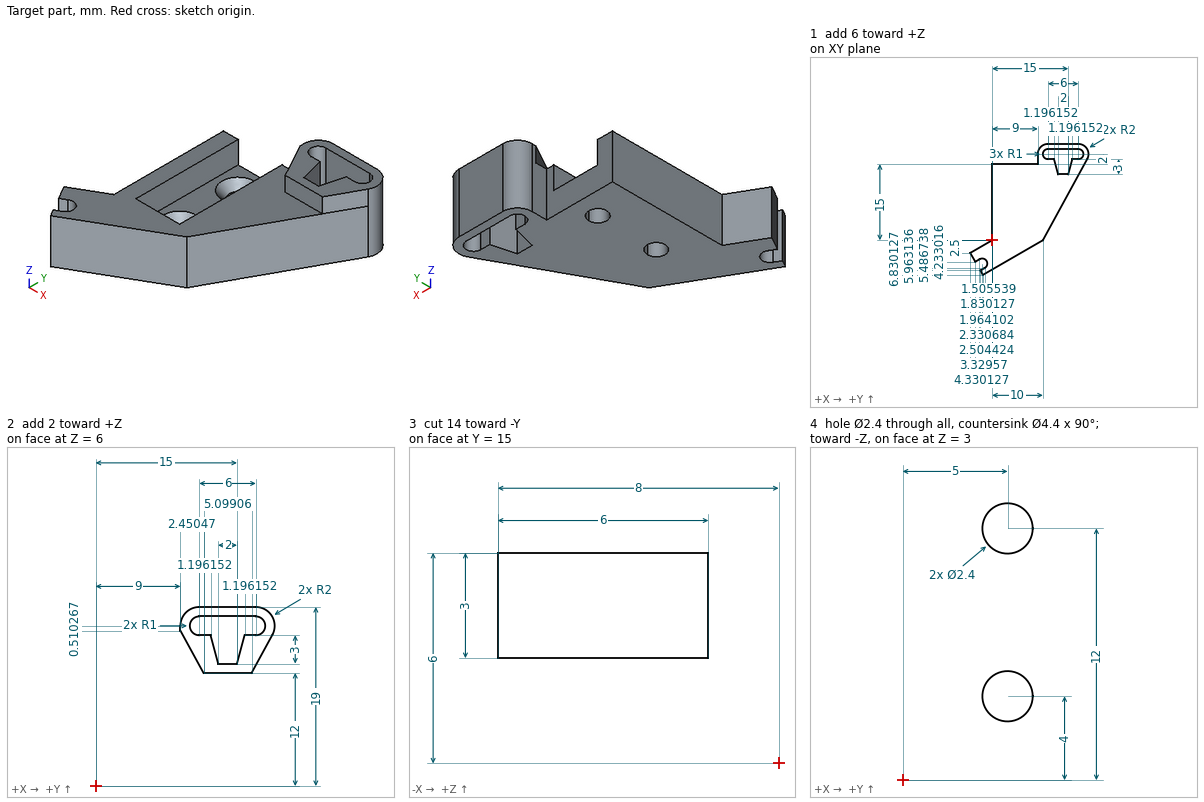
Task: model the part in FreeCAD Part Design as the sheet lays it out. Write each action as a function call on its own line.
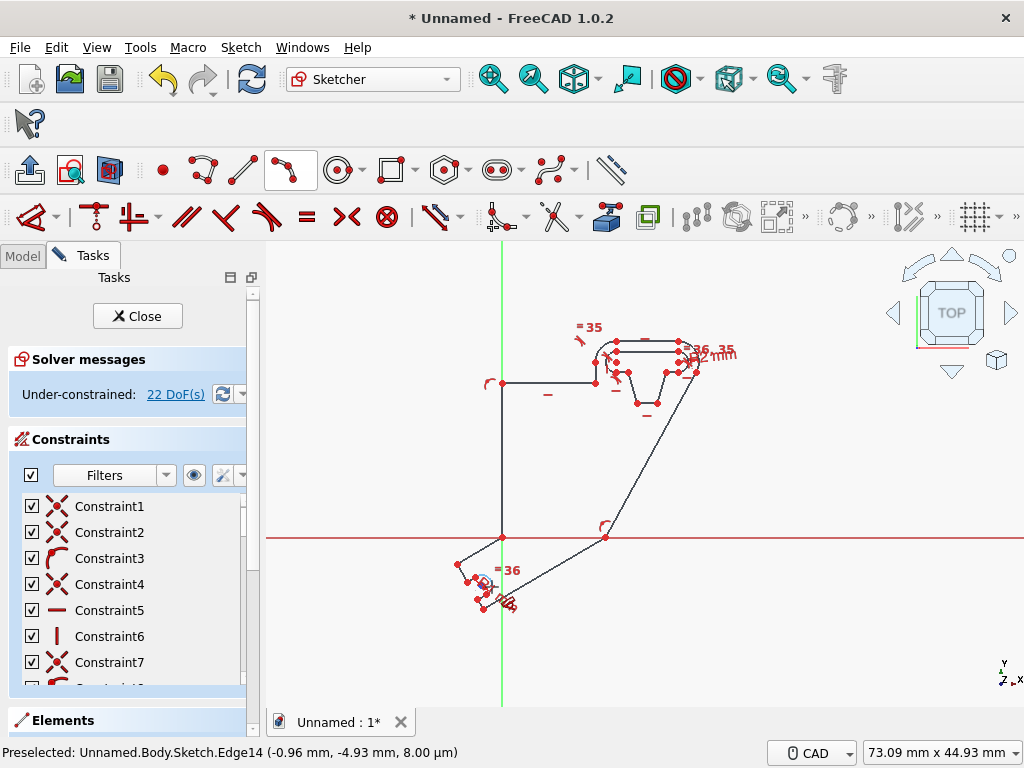
scroll(660, 341, up, 2)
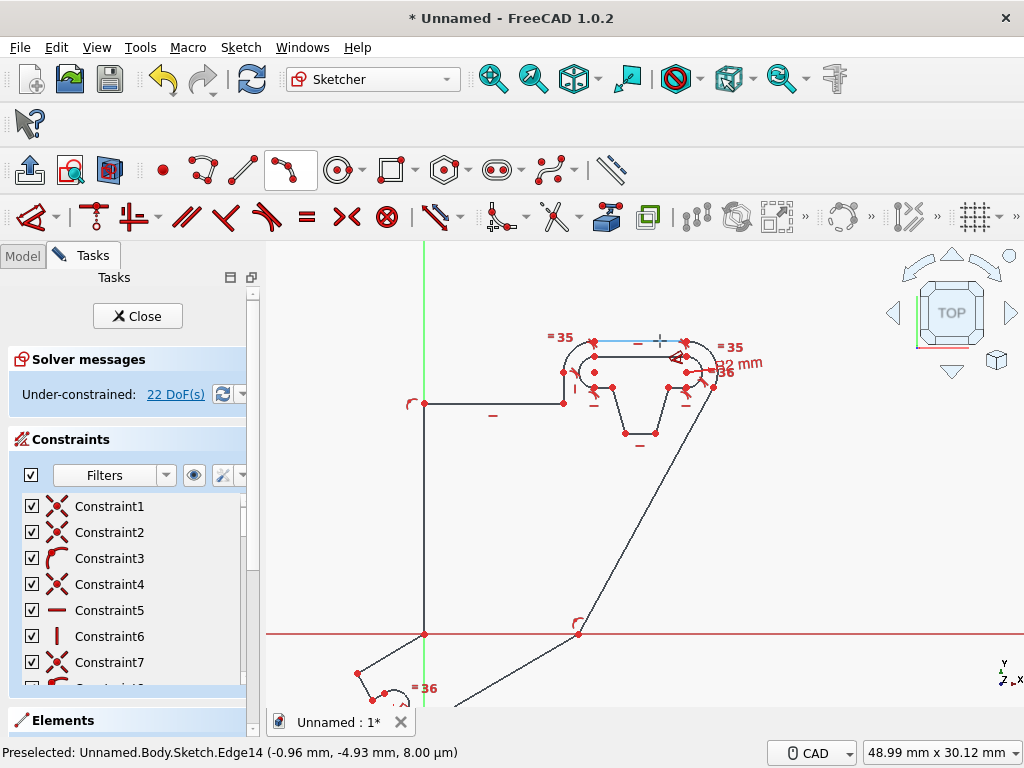
click(659, 341)
click(641, 307)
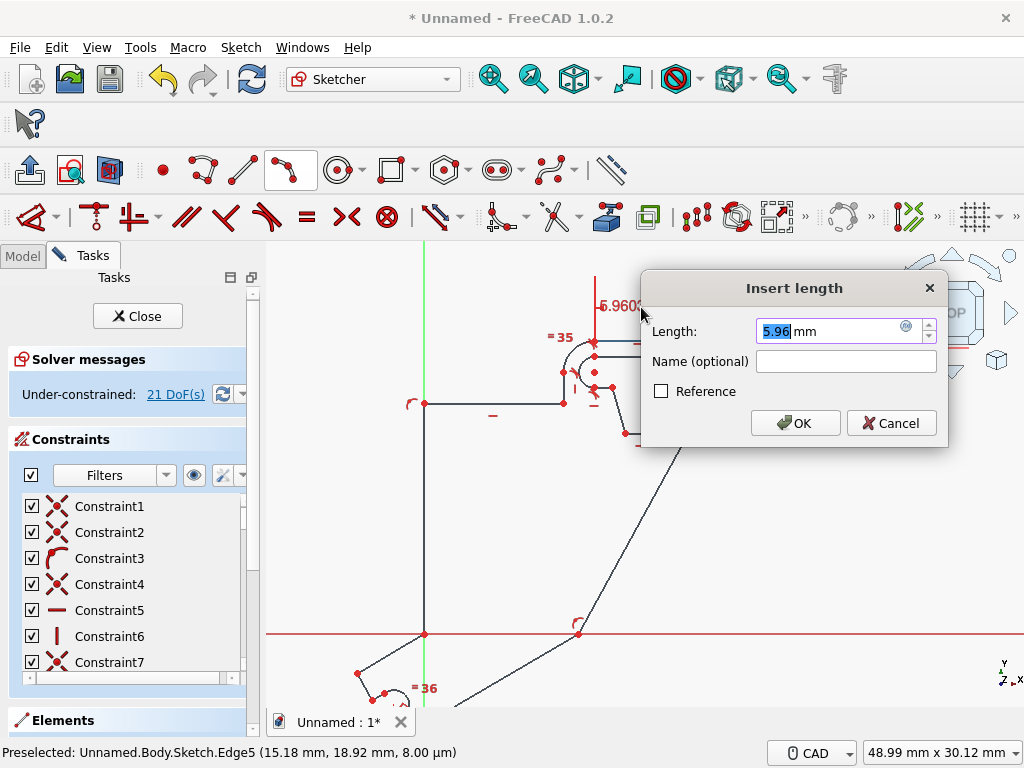
text(6)
key(Return)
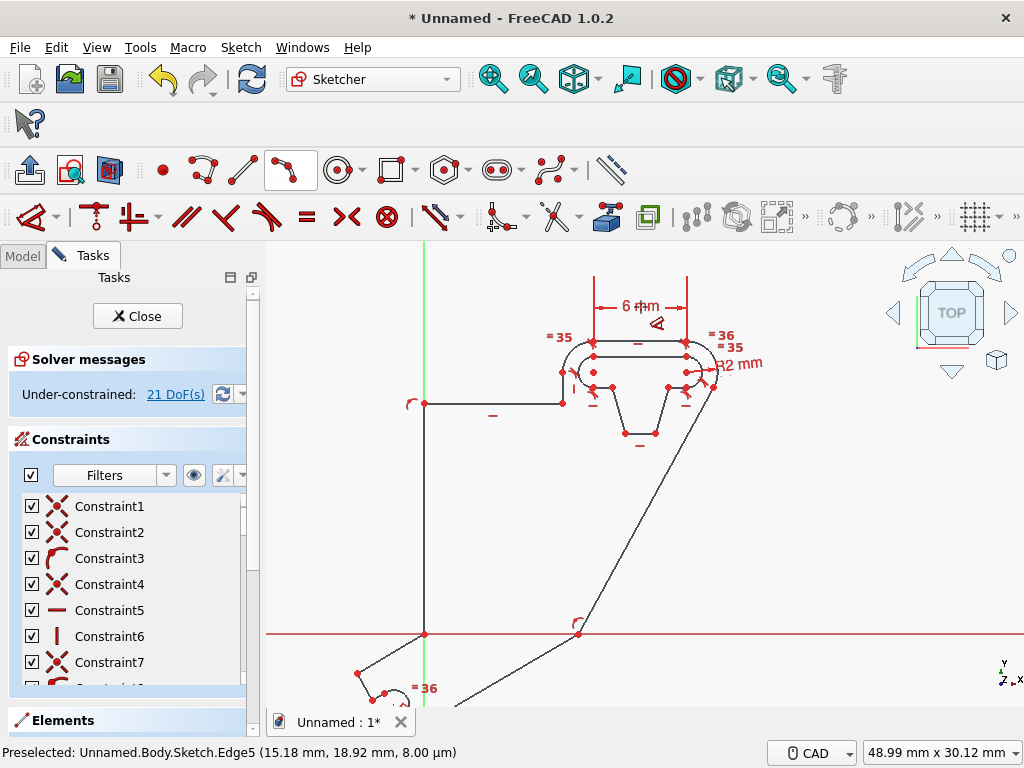
scroll(563, 382, up, 2)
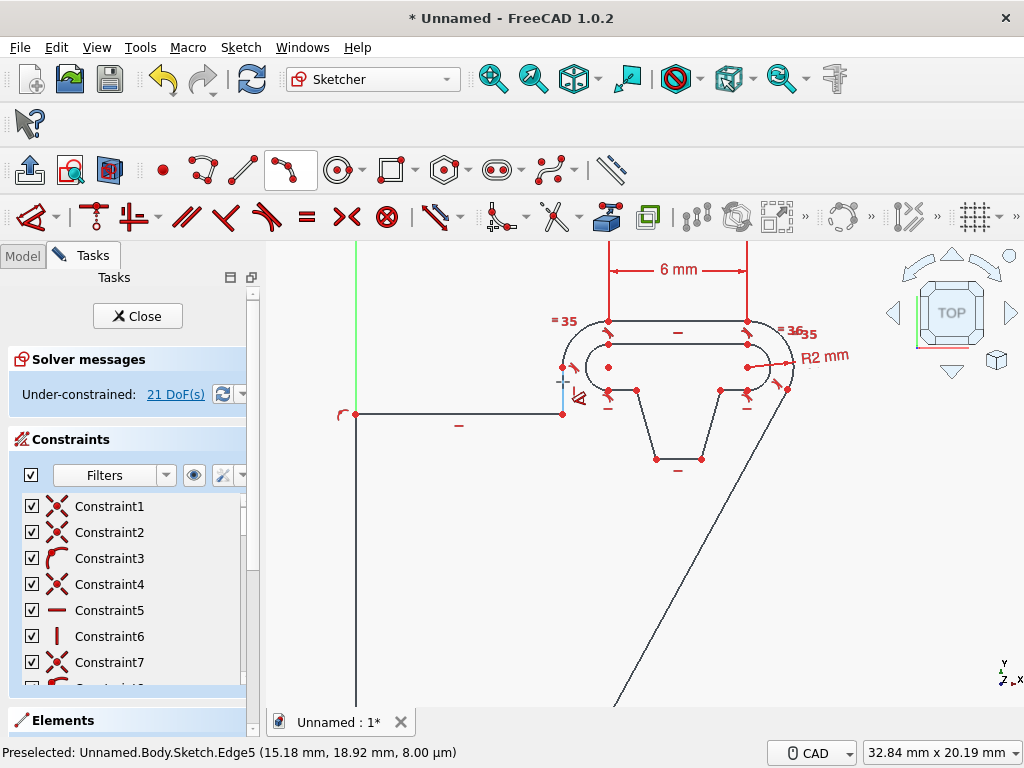
click(563, 381)
click(597, 402)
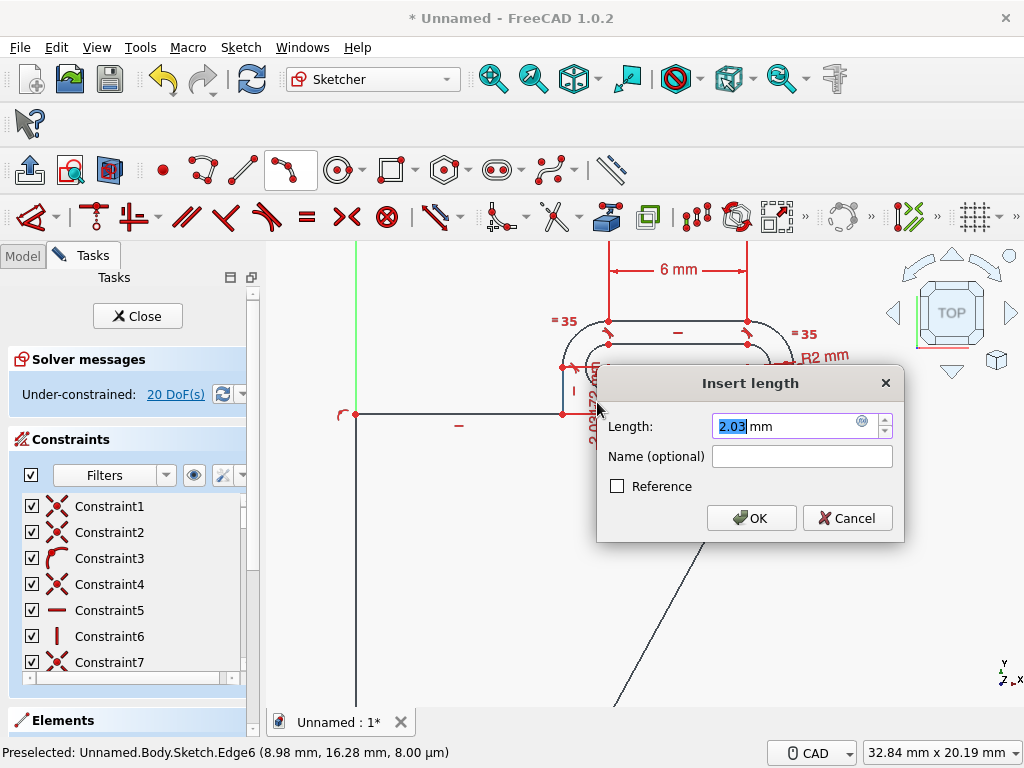
text(2)
key(Return)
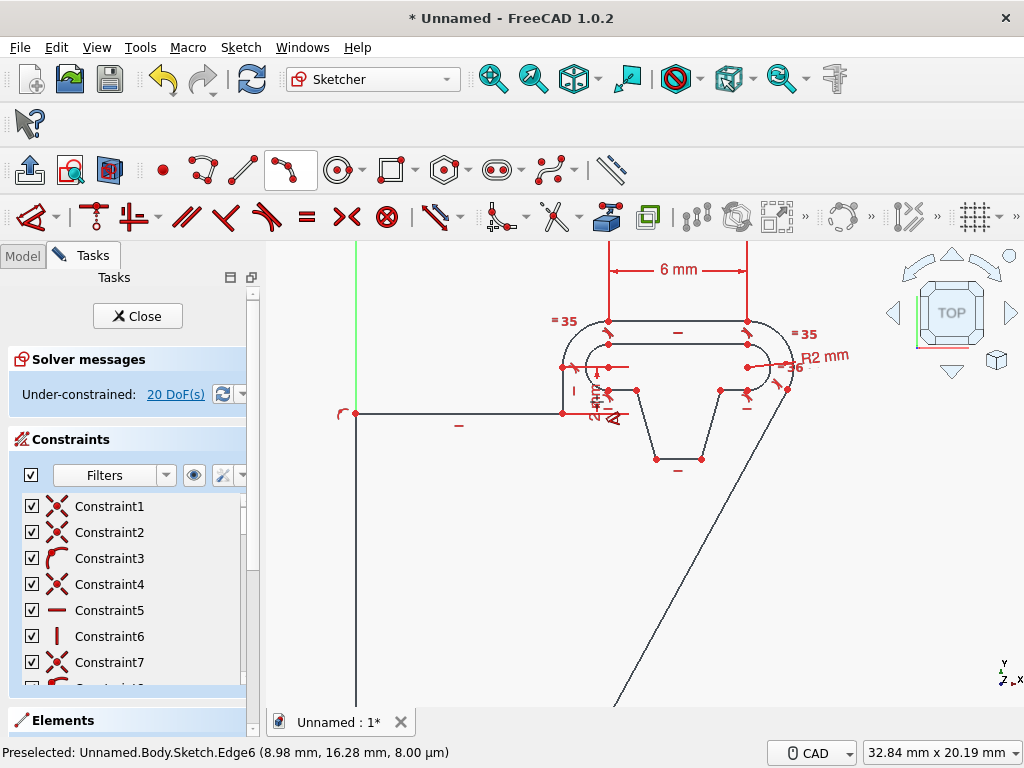
click(501, 414)
click(459, 380)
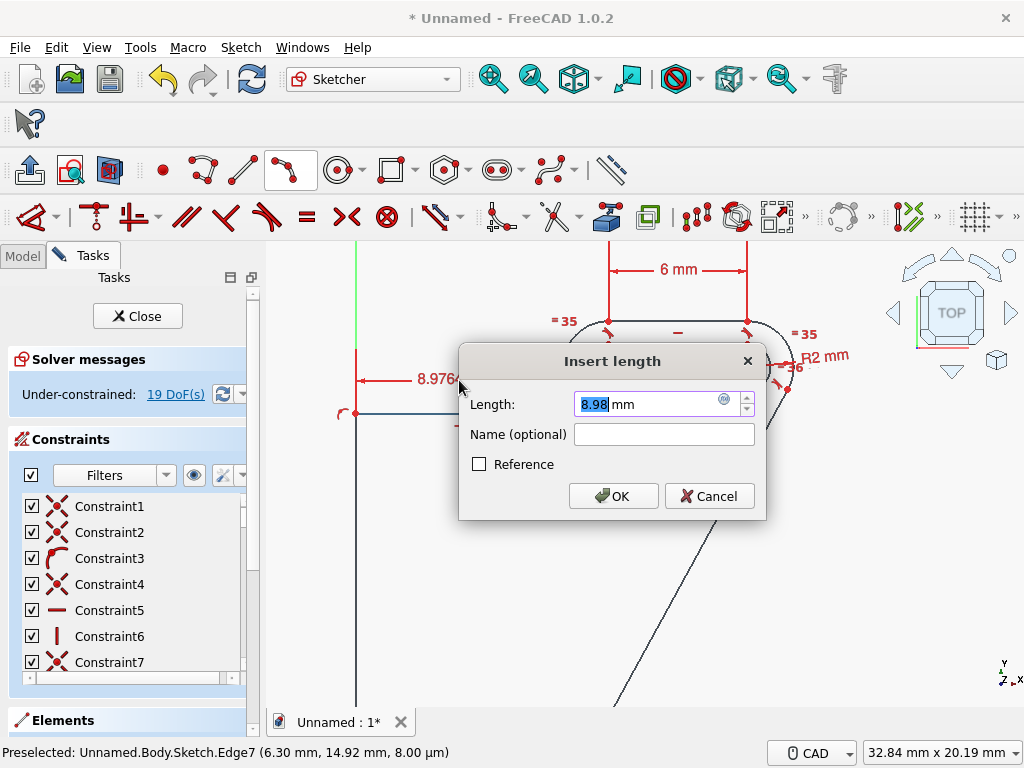
text(9)
key(Return)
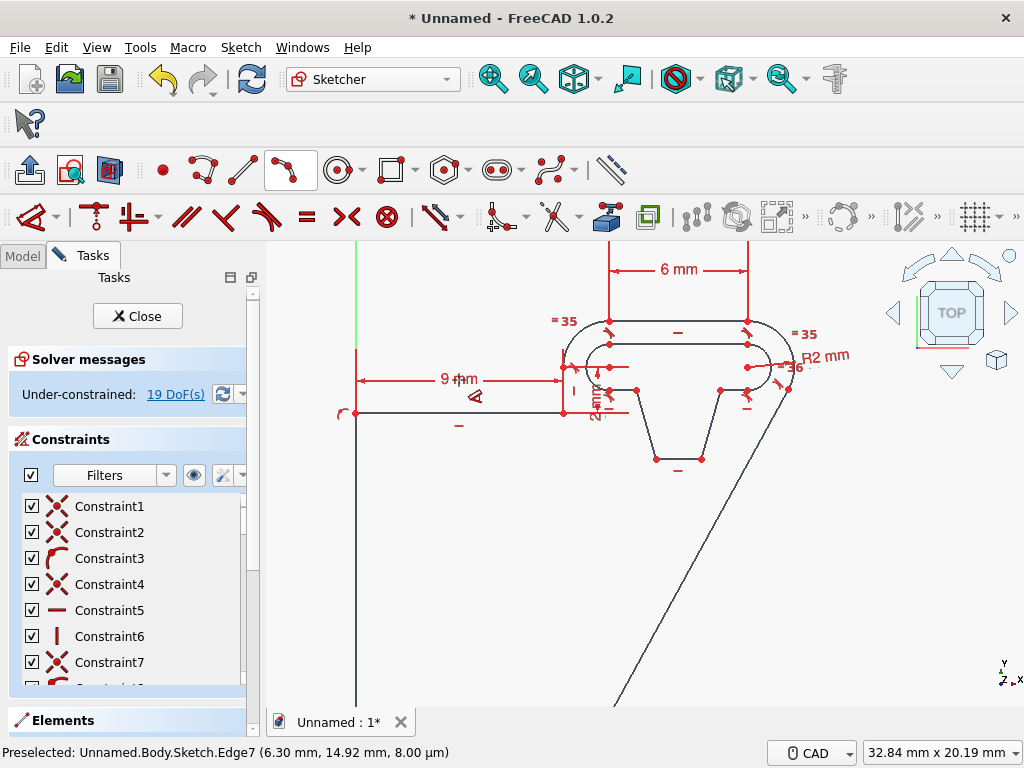
click(688, 459)
click(679, 425)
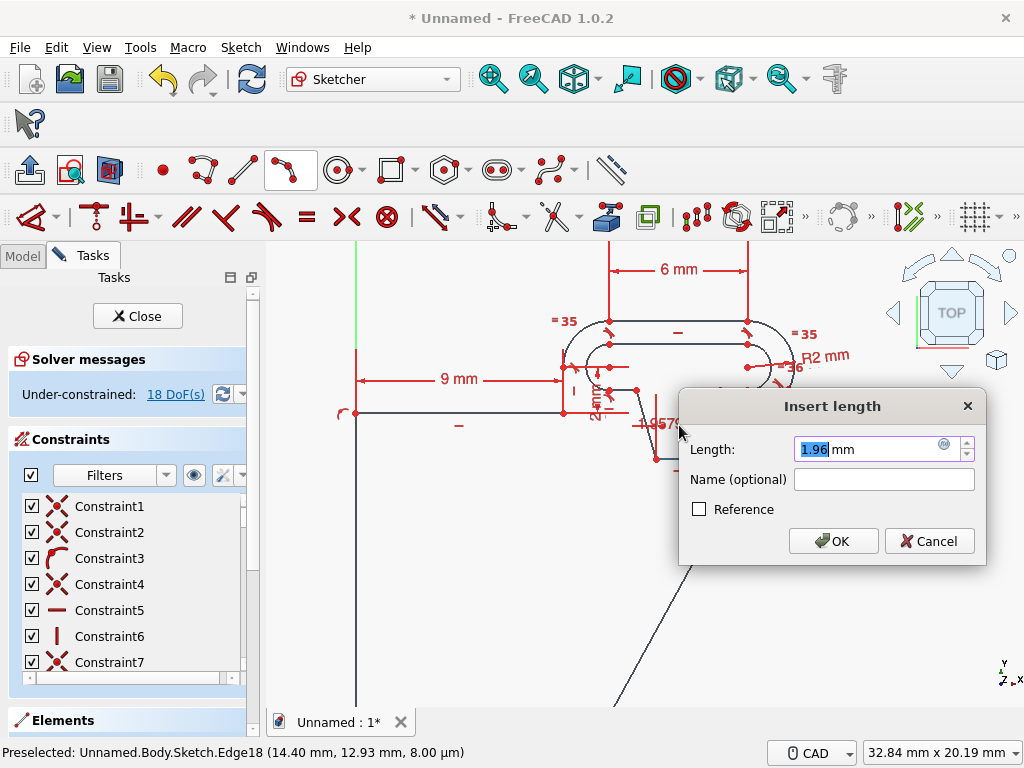
text(2)
key(Return)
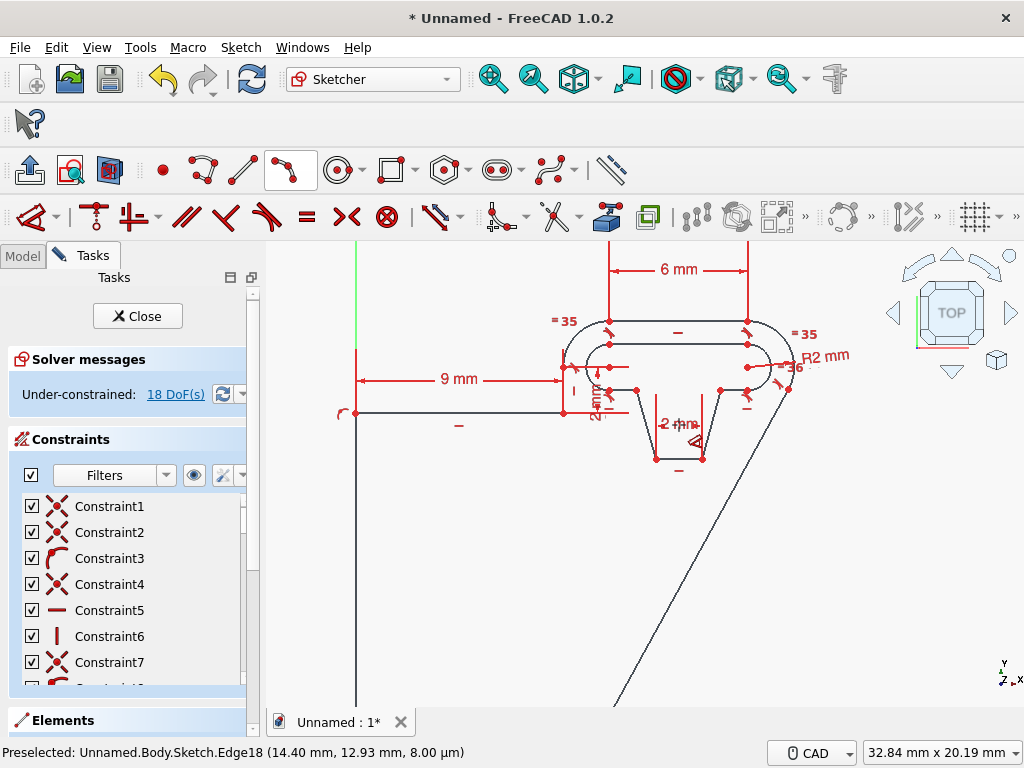
click(356, 517)
click(322, 546)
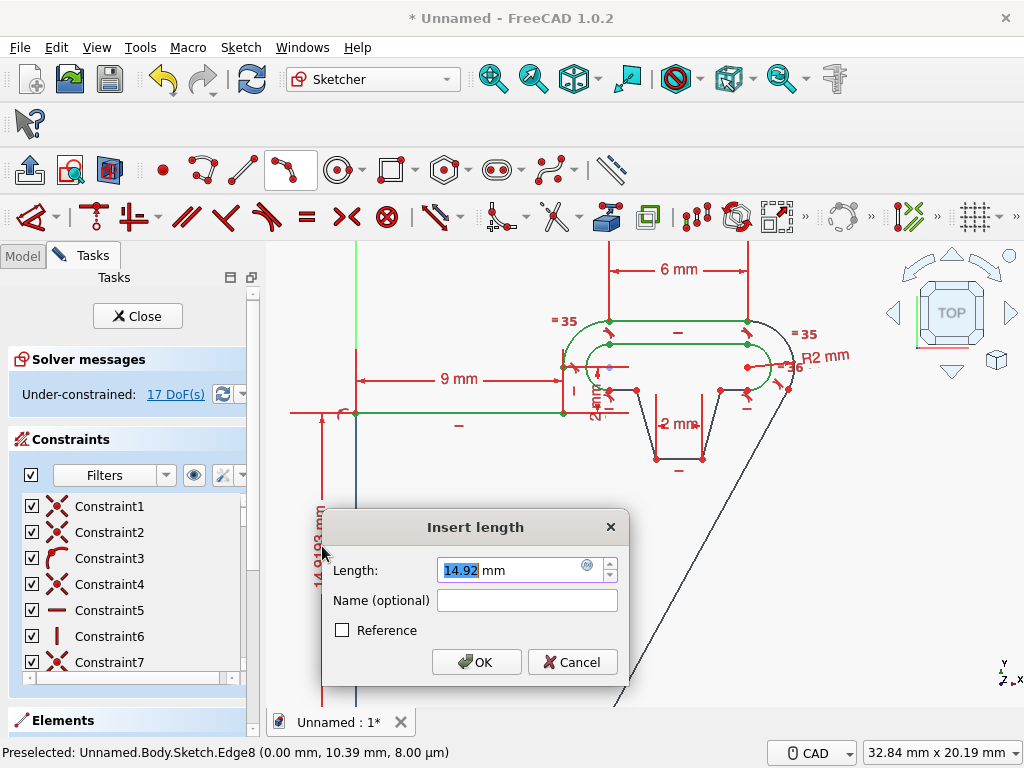
text(15)
key(Return)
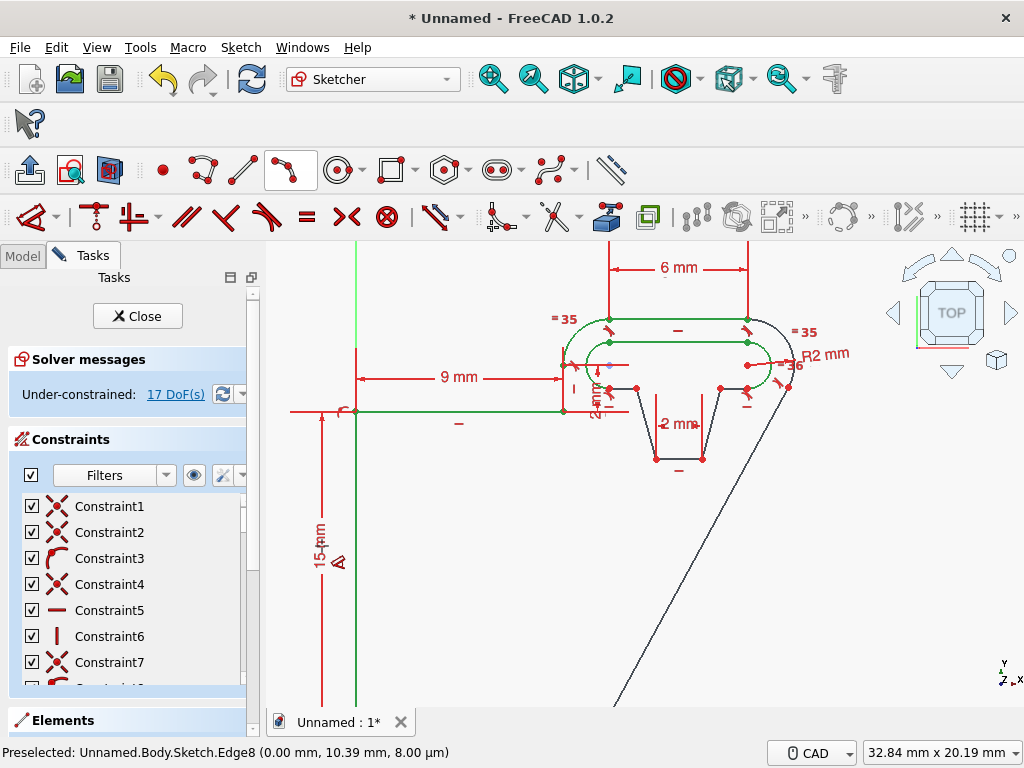
click(715, 410)
click(755, 408)